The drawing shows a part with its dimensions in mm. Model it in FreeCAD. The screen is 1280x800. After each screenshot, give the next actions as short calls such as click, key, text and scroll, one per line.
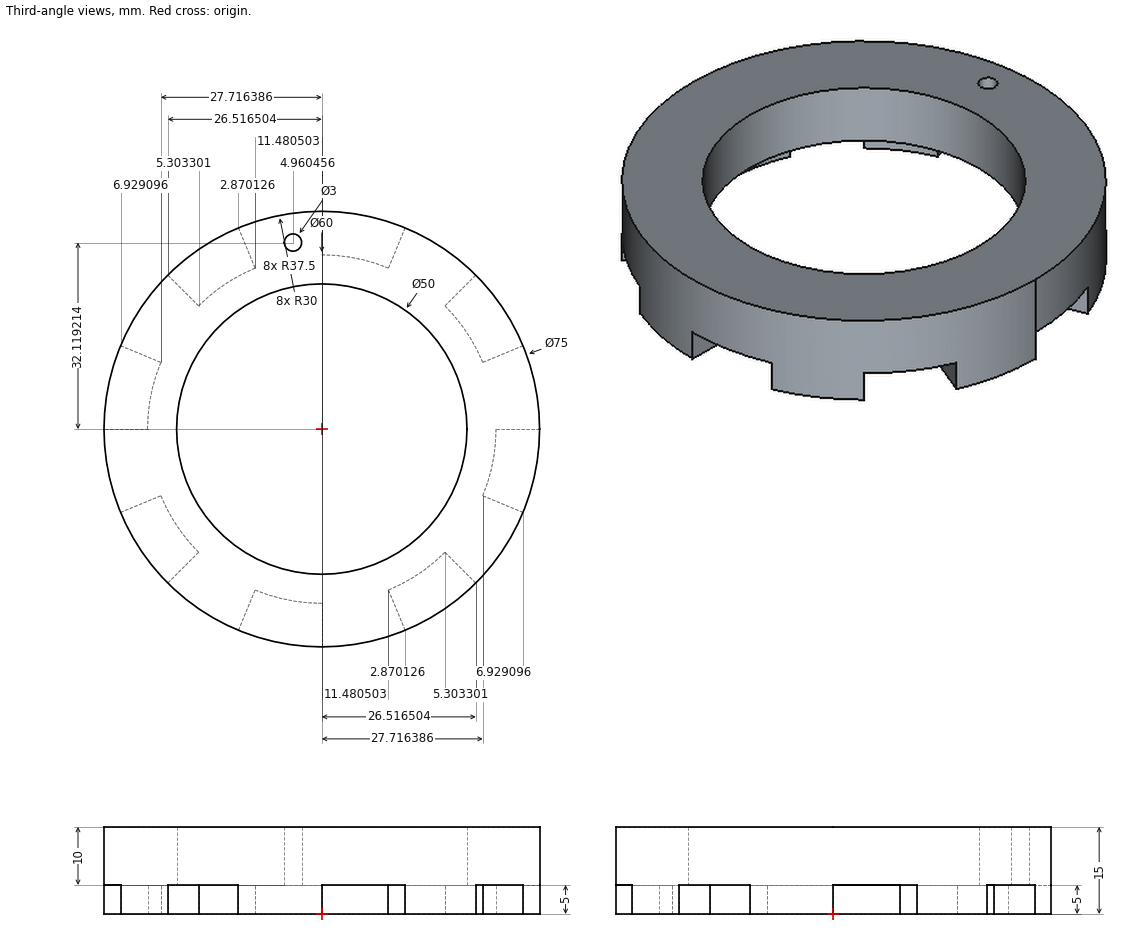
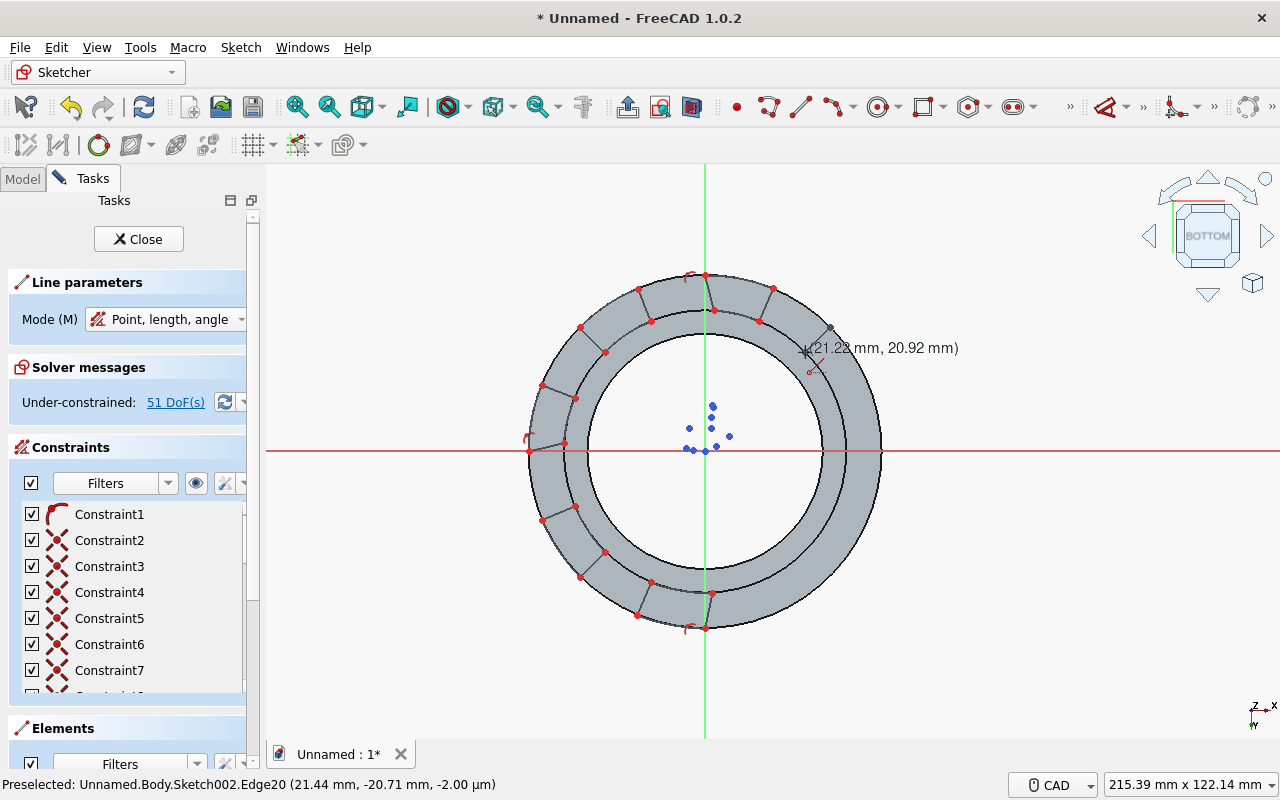
click(836, 397)
click(868, 384)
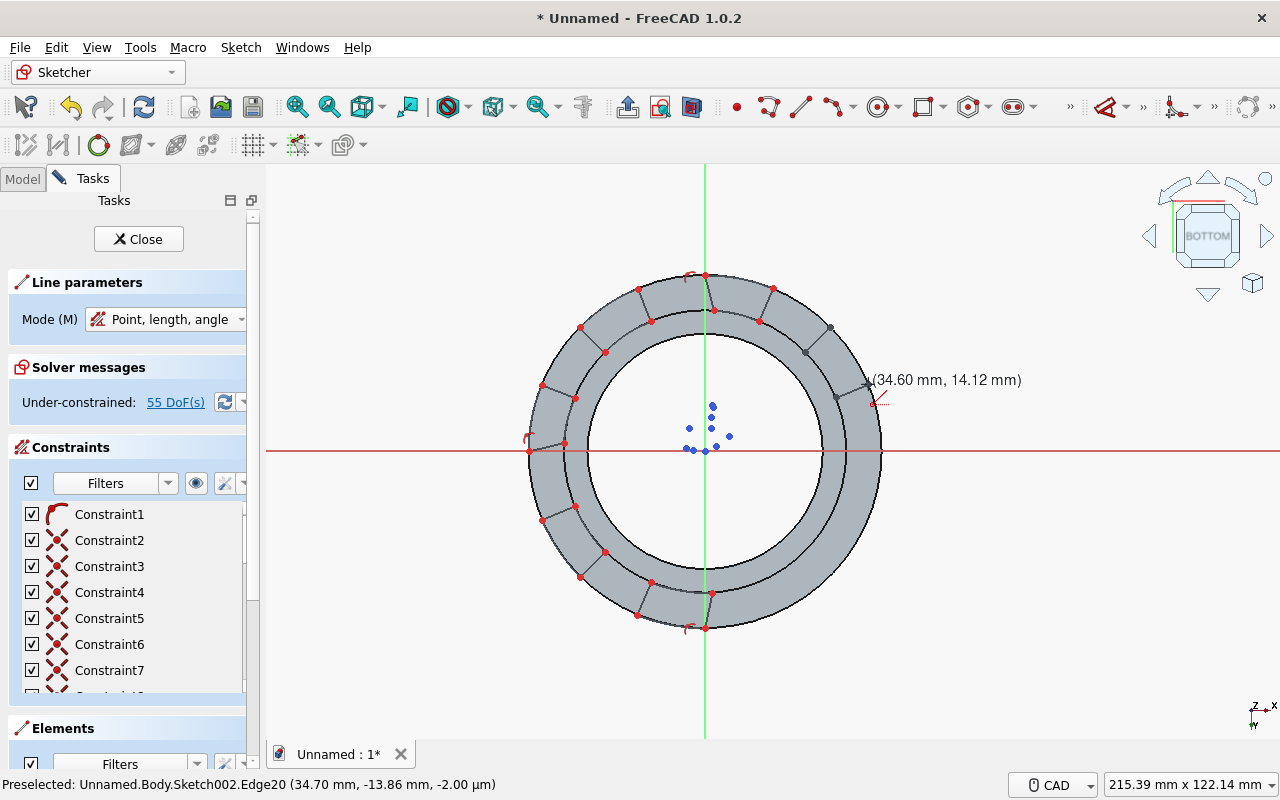
key(g)
key(3)
key(a)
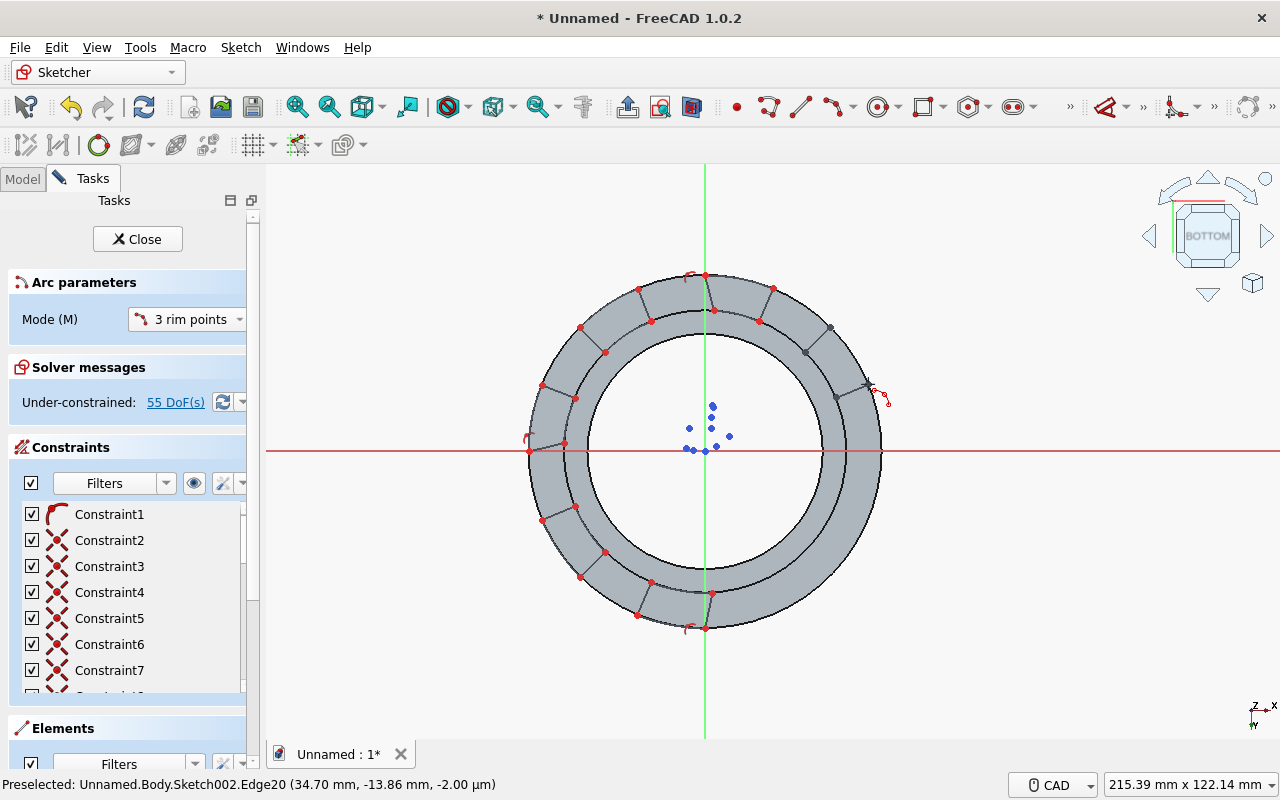
click(805, 353)
click(836, 398)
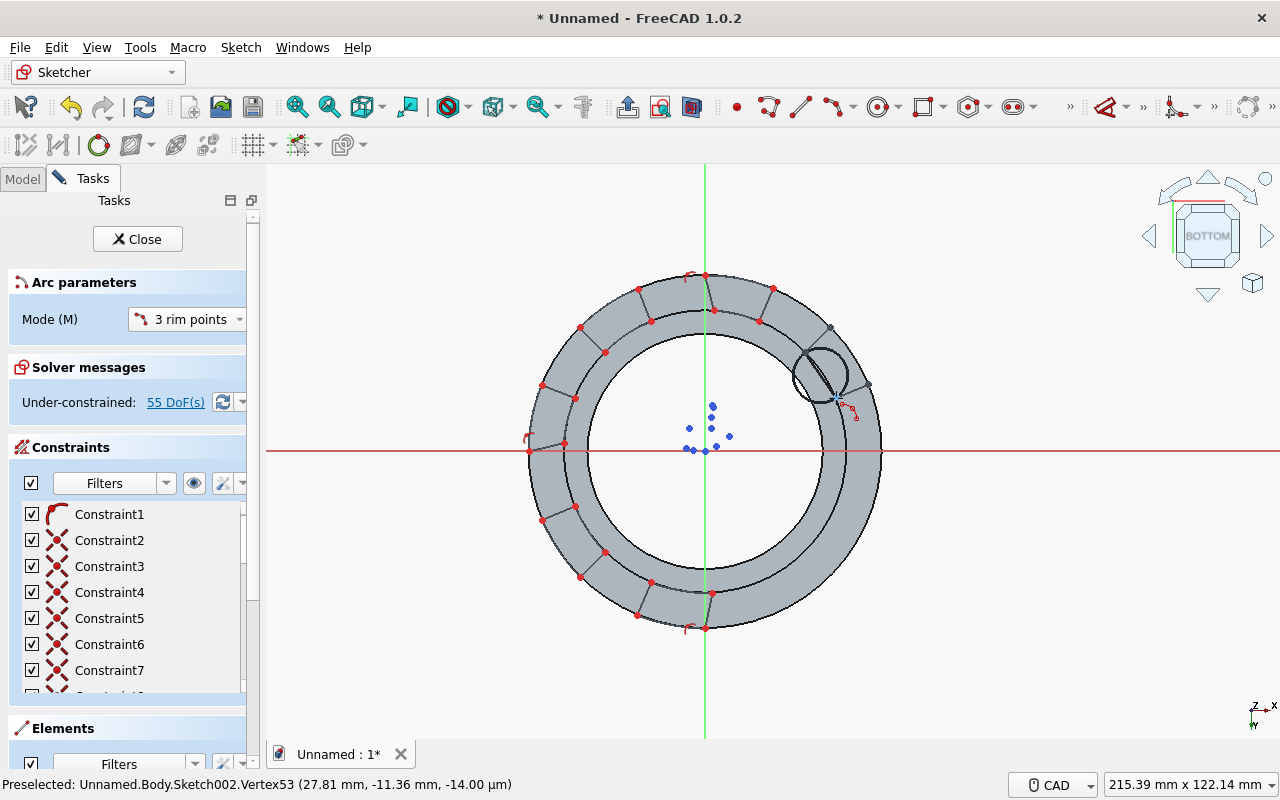
scroll(823, 373, up, 9)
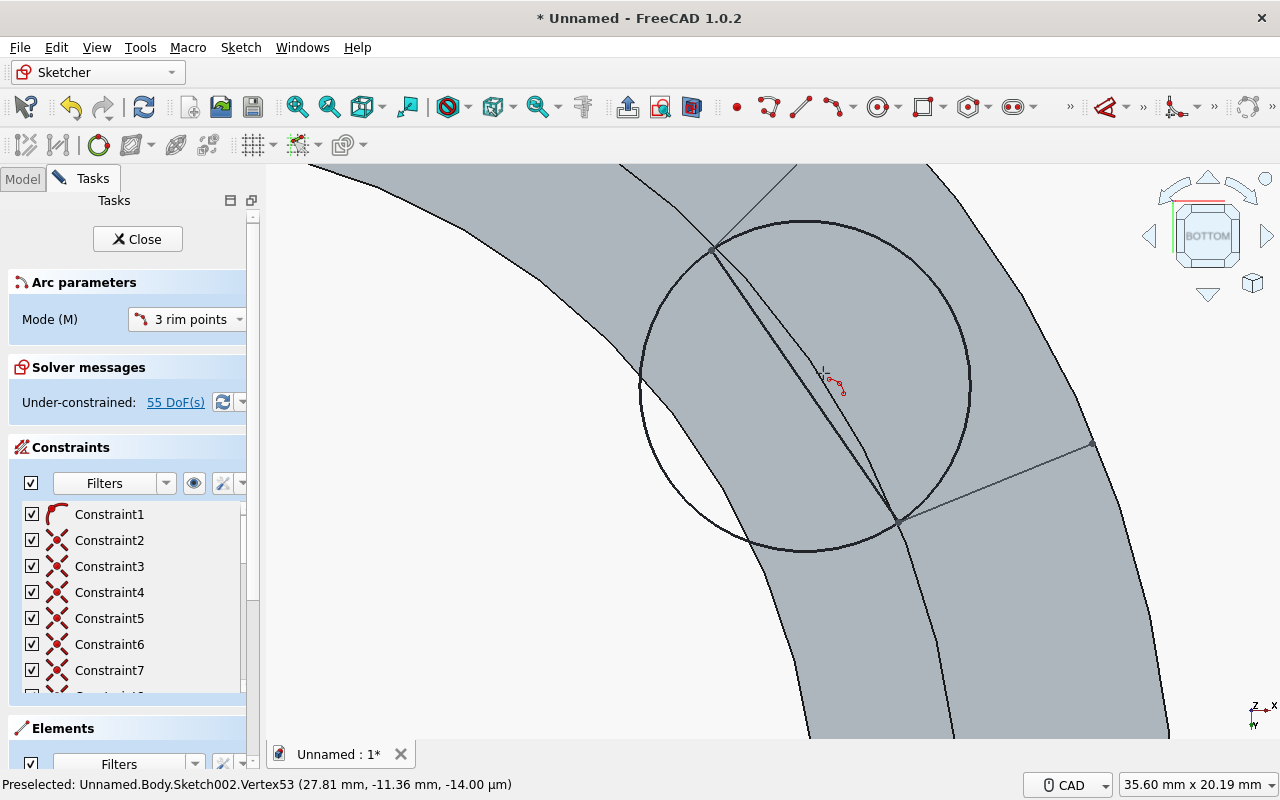
click(817, 371)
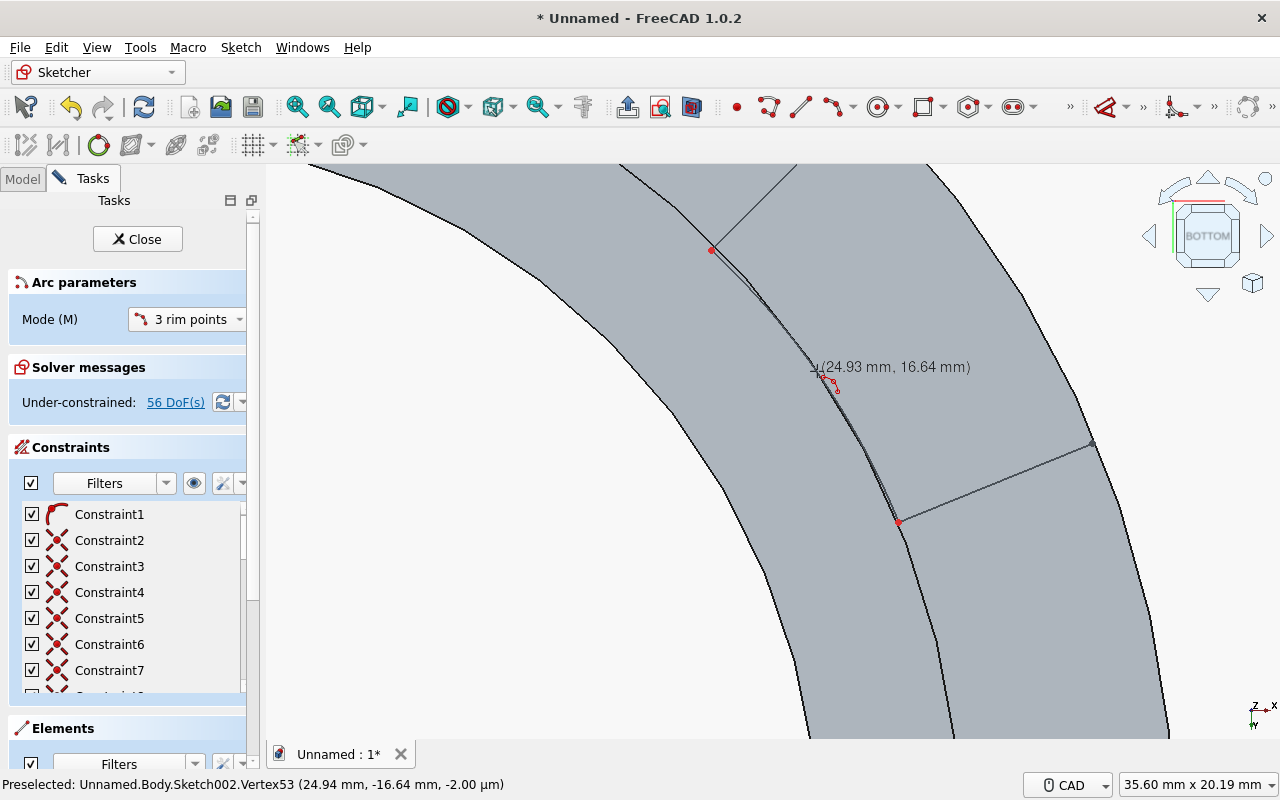
scroll(823, 373, down, 9)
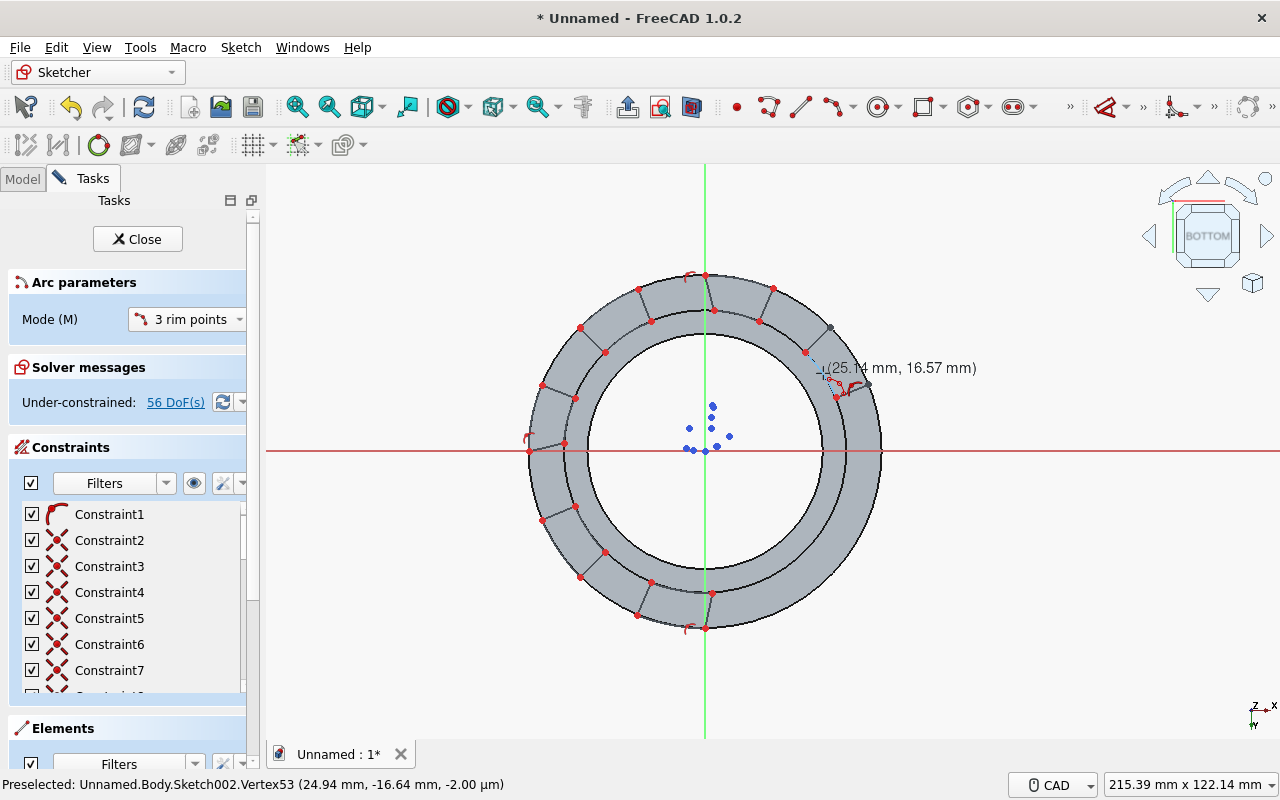
click(868, 385)
click(830, 328)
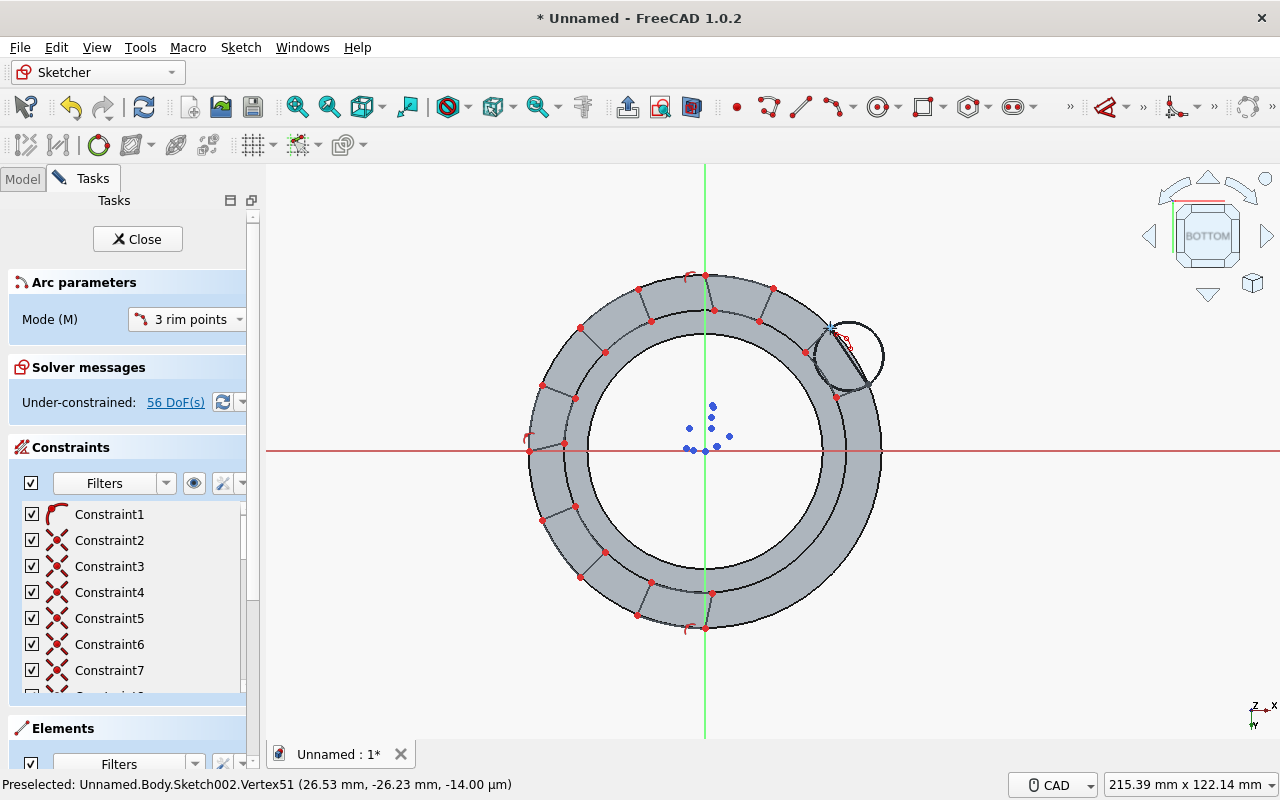
scroll(852, 353, up, 8)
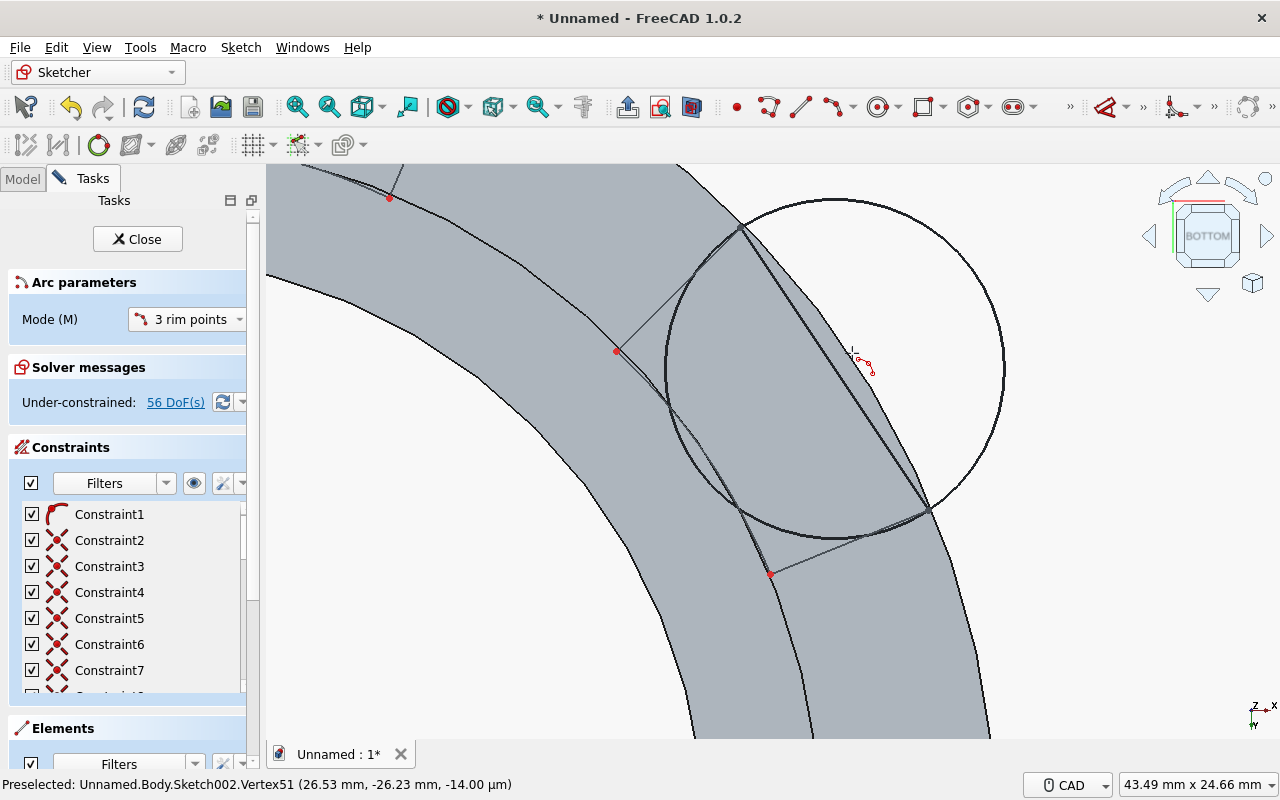
click(849, 354)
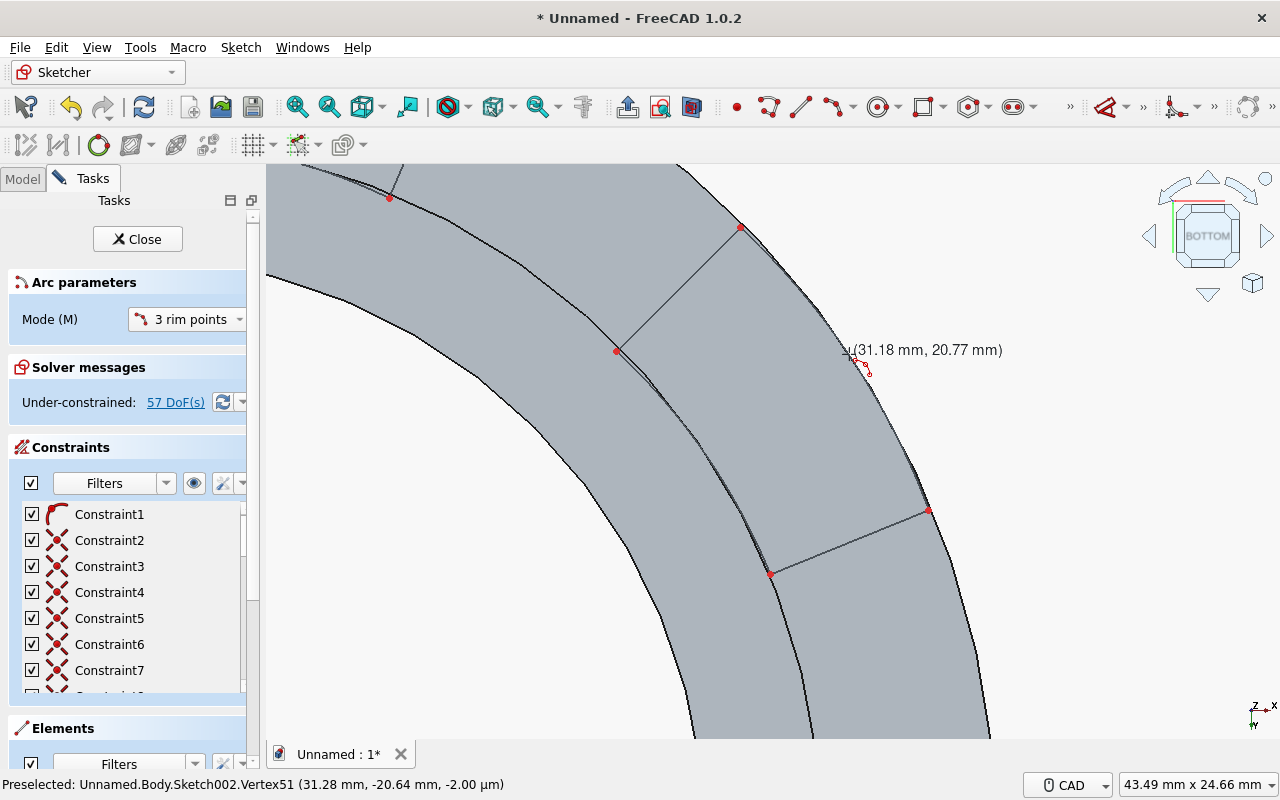
click(802, 108)